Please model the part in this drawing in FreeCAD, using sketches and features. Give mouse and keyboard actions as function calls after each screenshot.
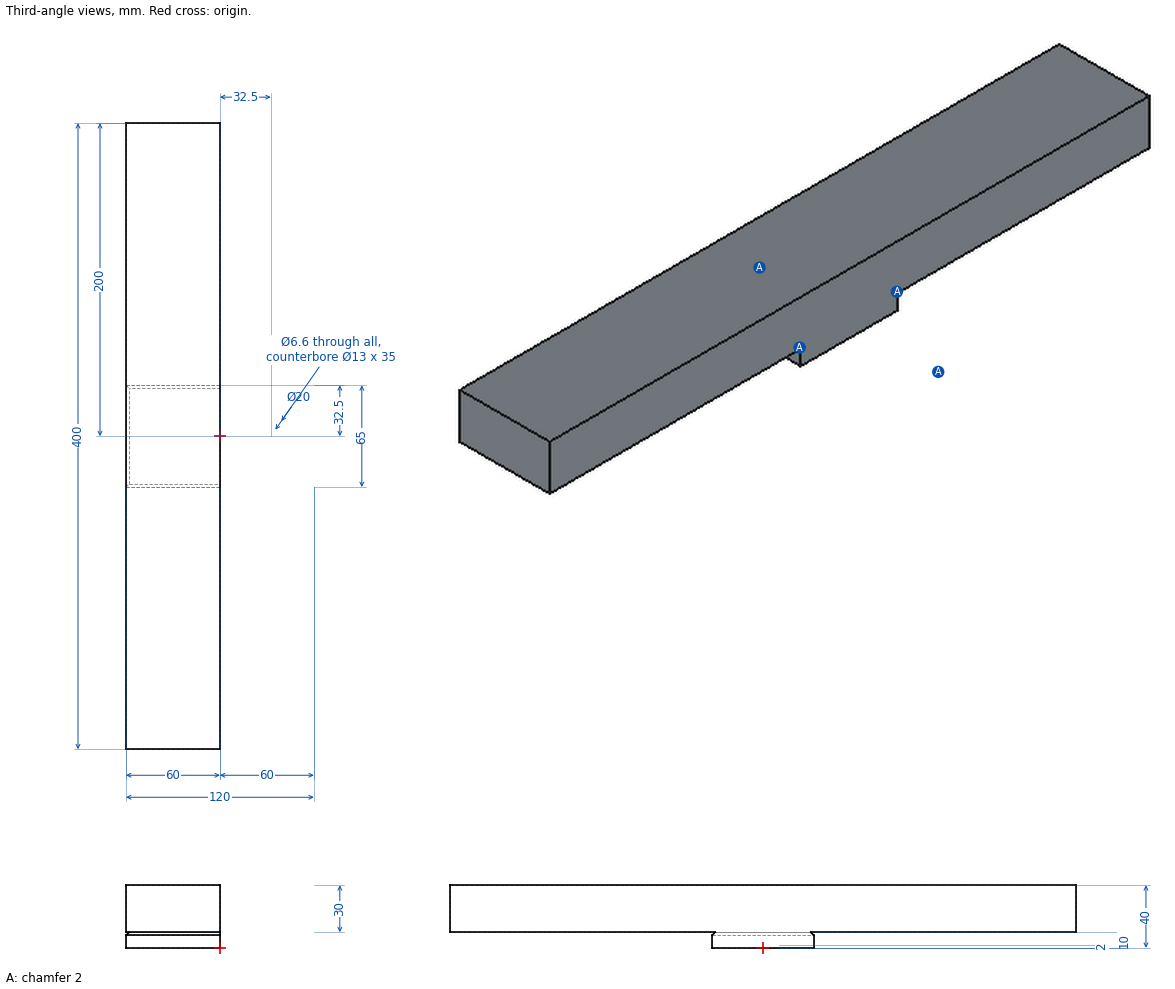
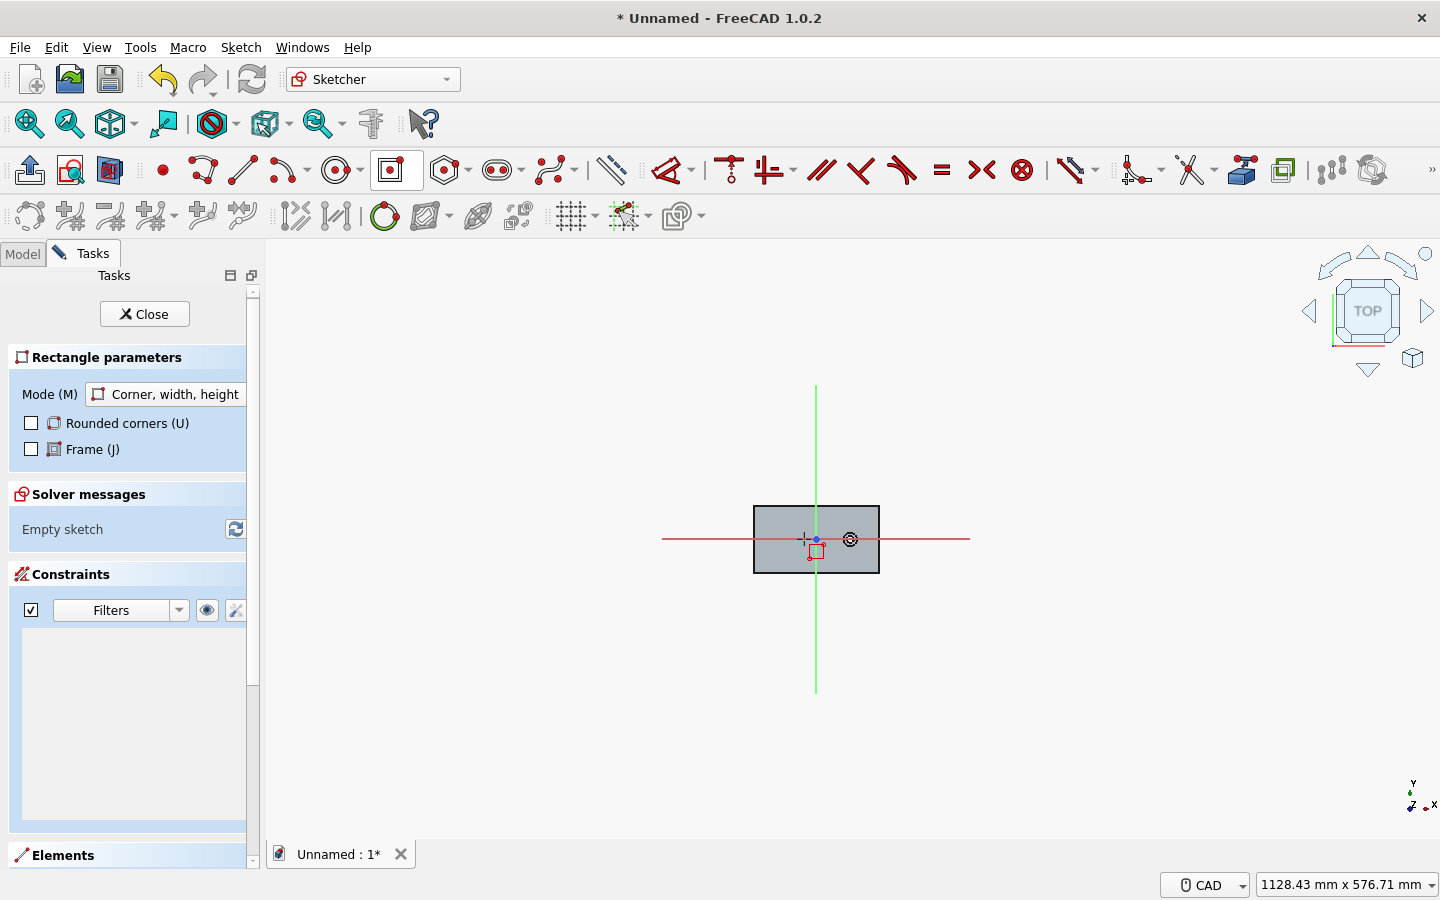
click(754, 331)
click(816, 747)
key(Escape)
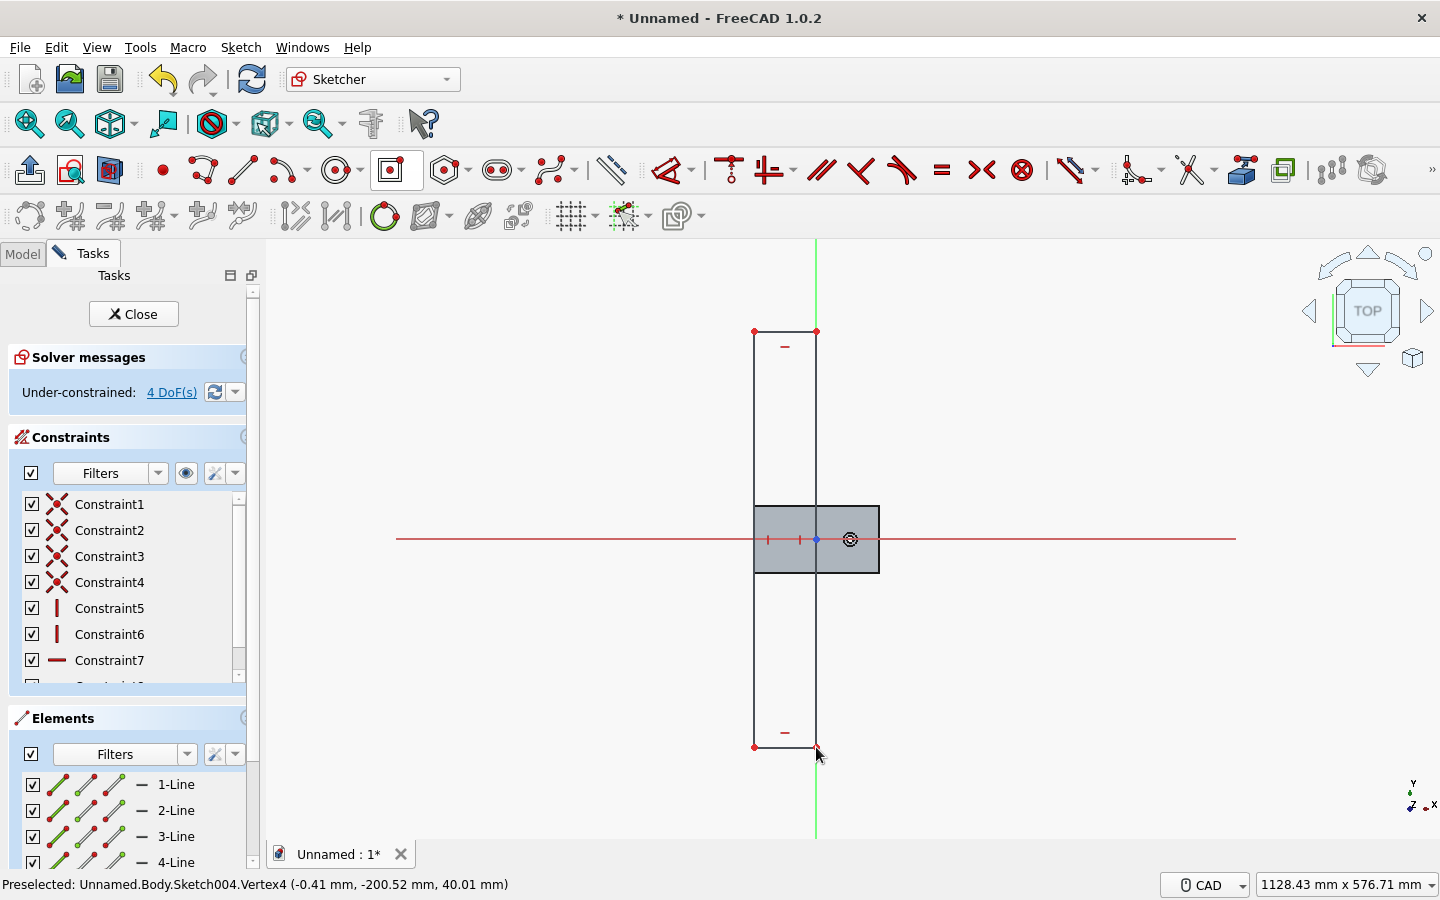
click(816, 748)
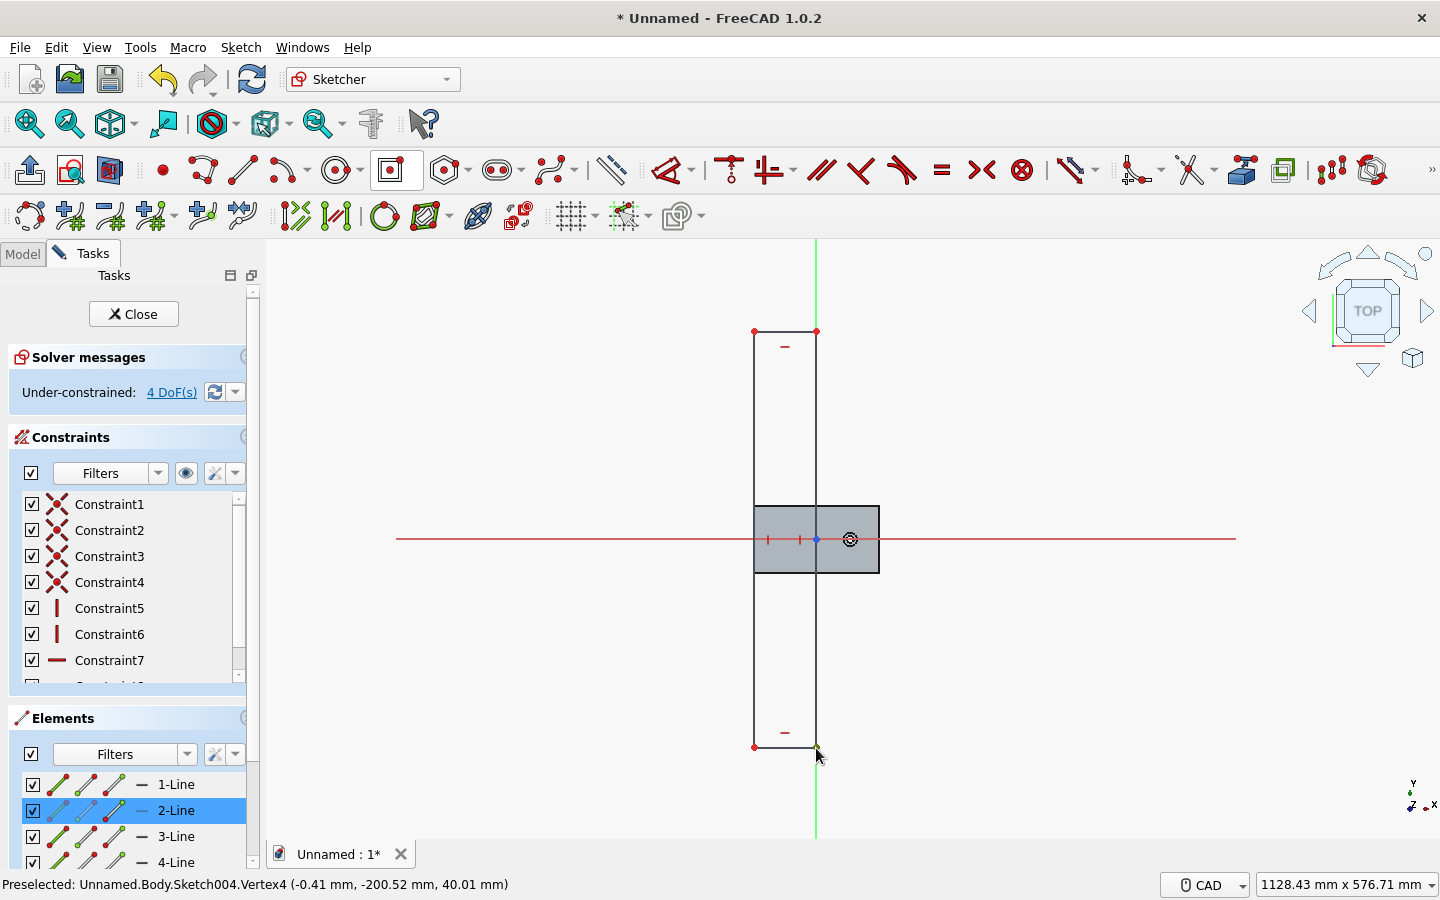
click(816, 306)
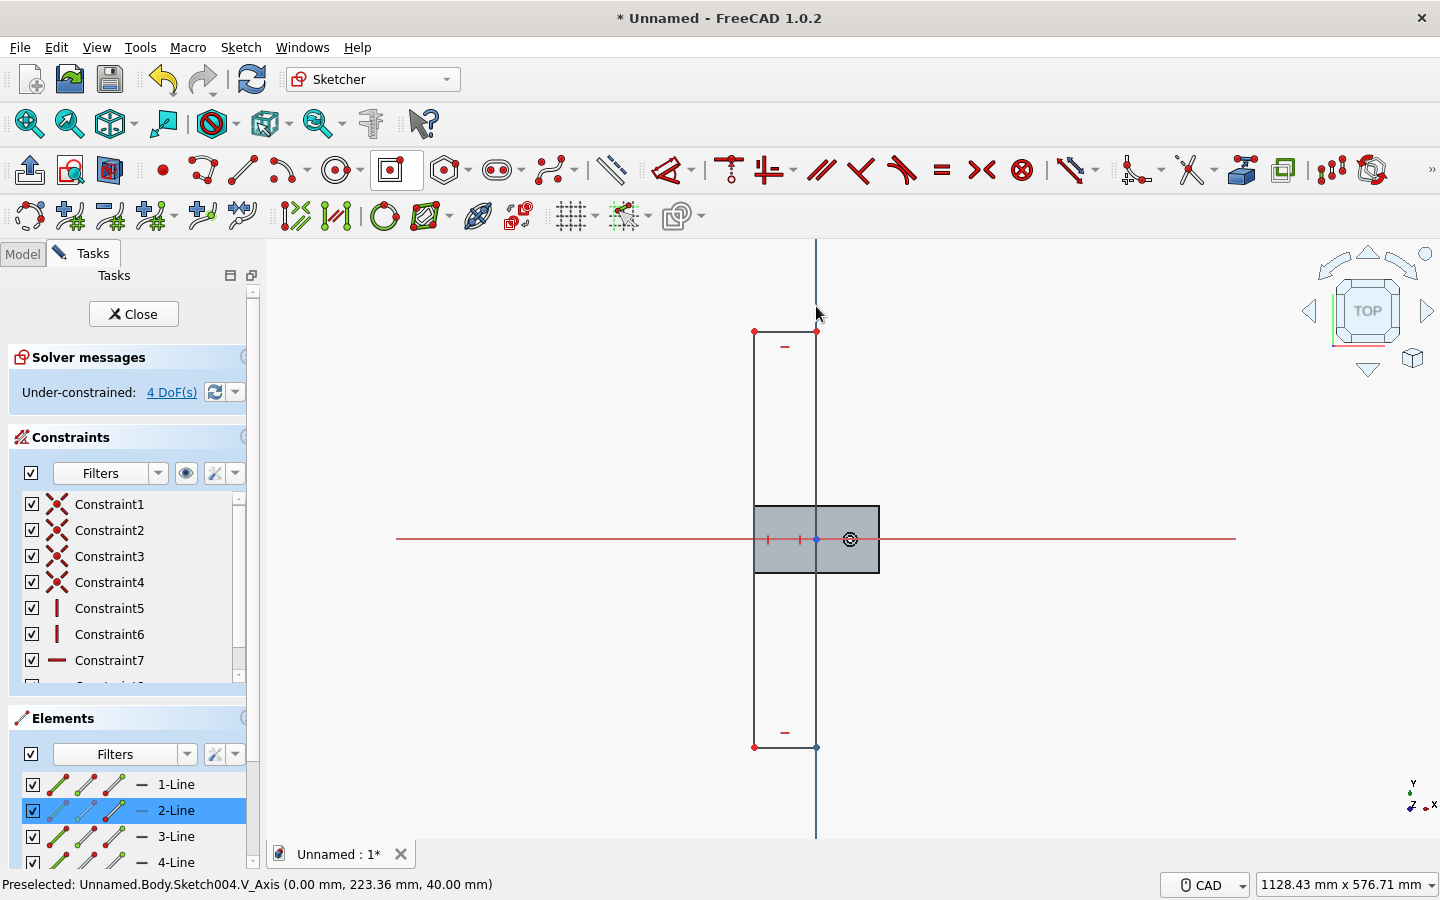
click(730, 170)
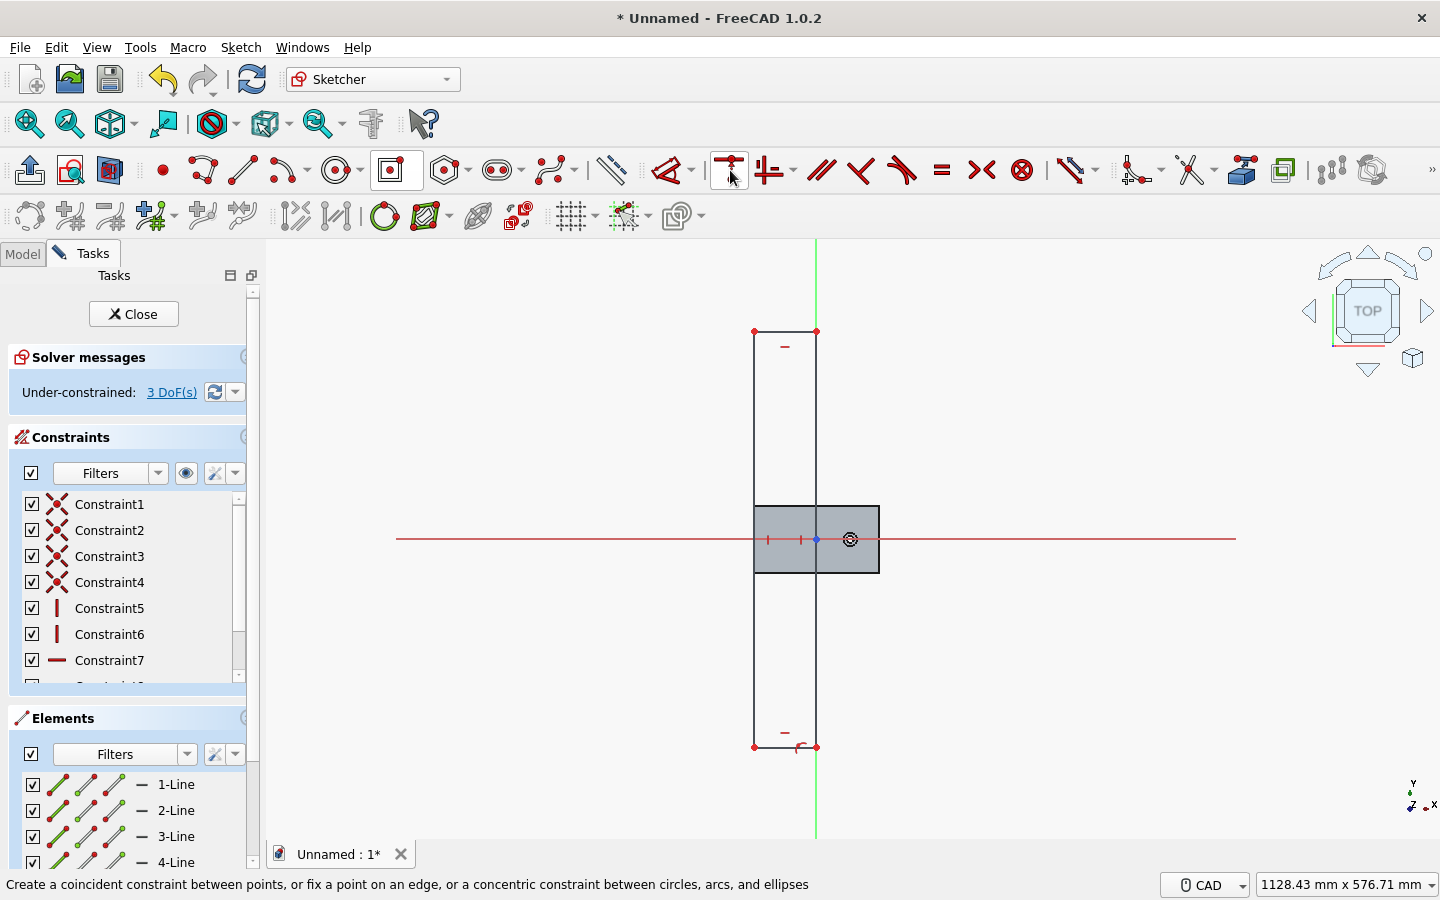
key(d)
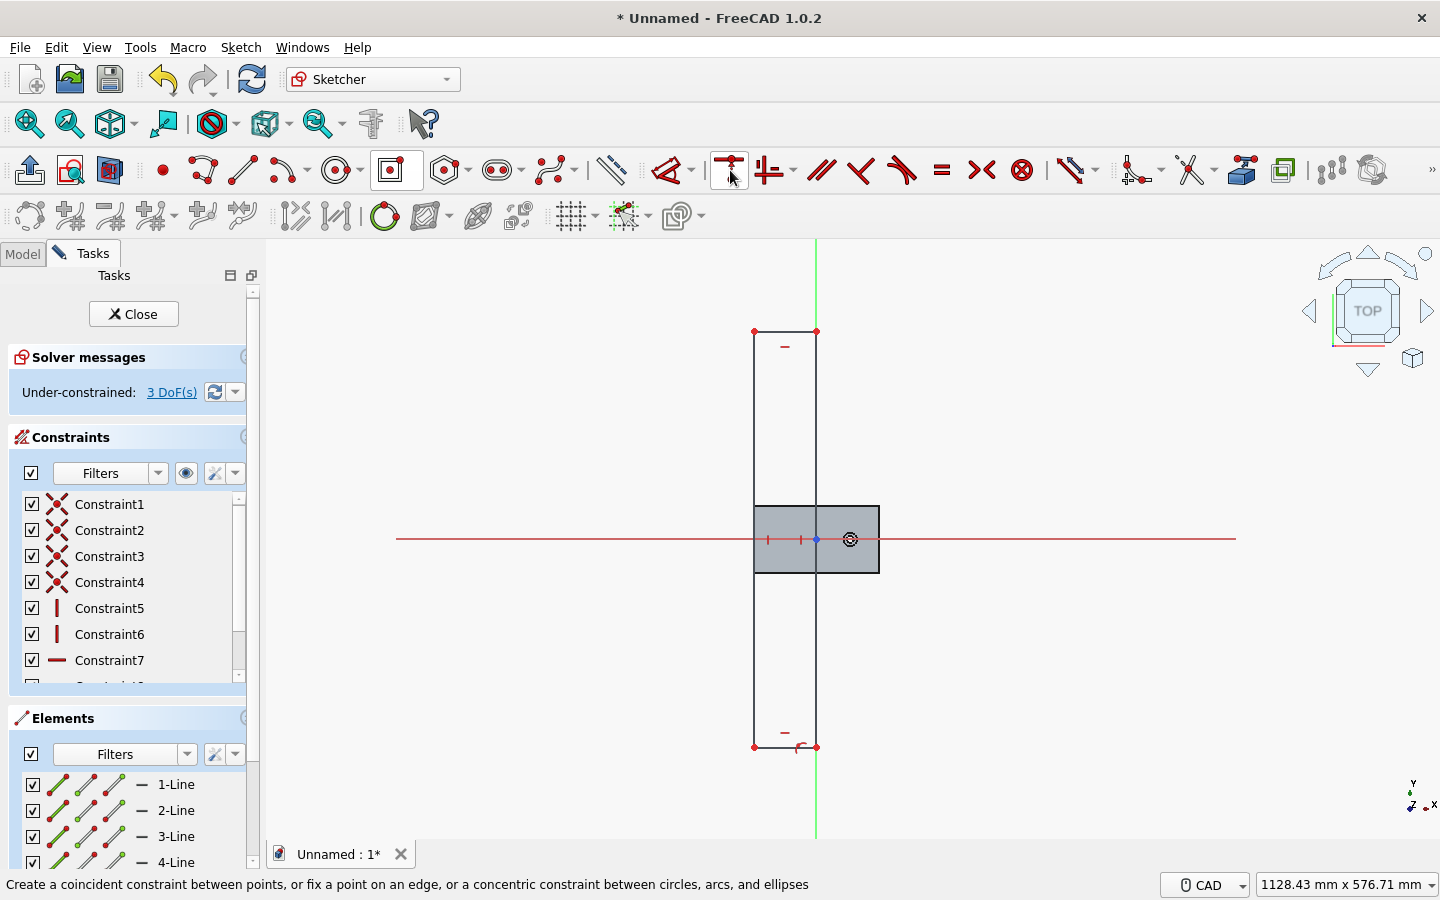
click(773, 748)
click(785, 782)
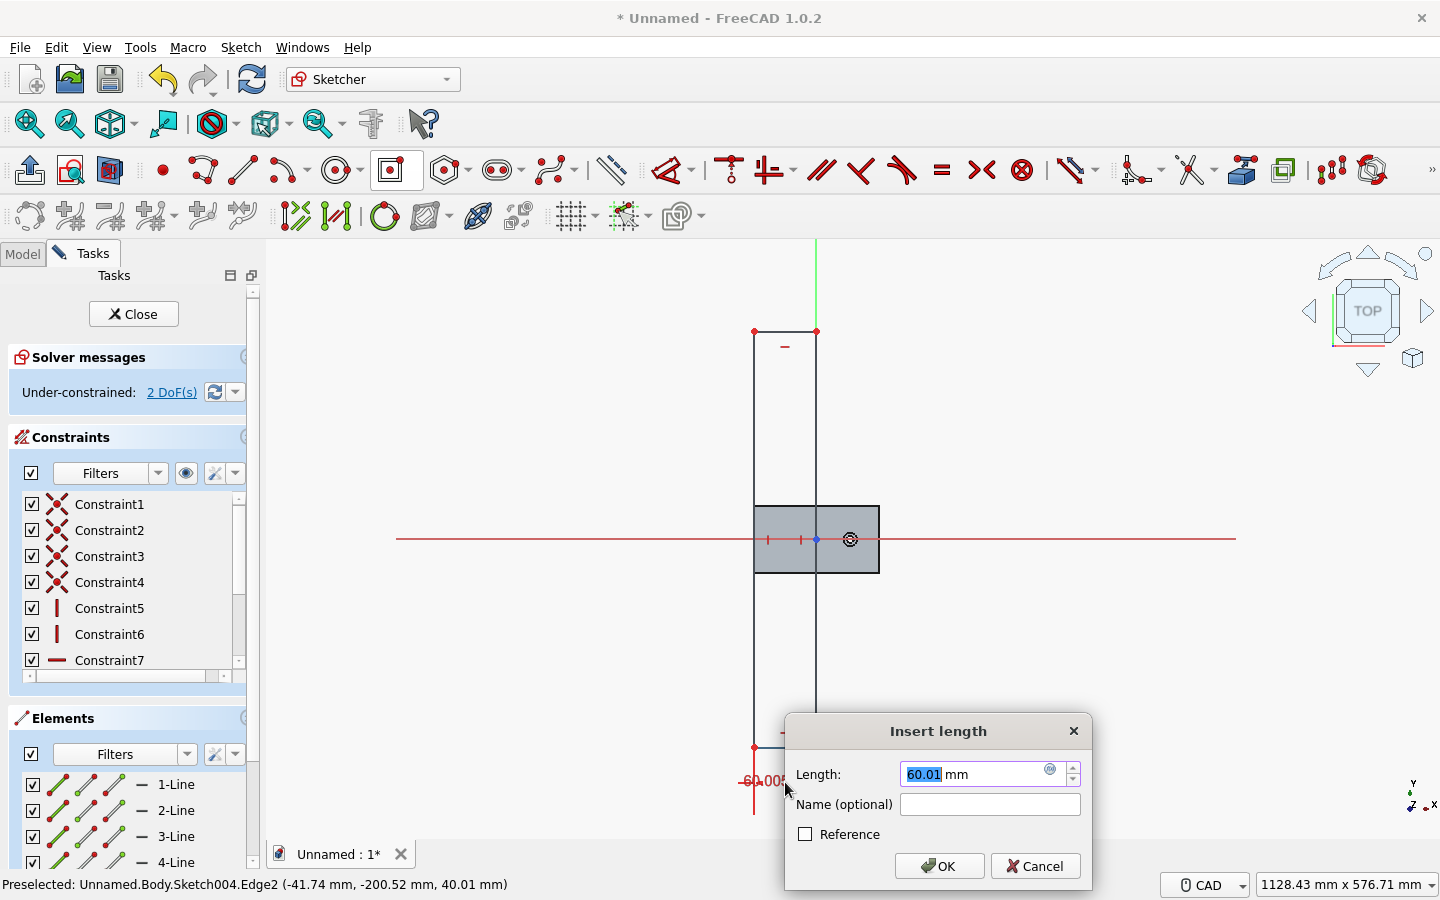
text(60)
key(Return)